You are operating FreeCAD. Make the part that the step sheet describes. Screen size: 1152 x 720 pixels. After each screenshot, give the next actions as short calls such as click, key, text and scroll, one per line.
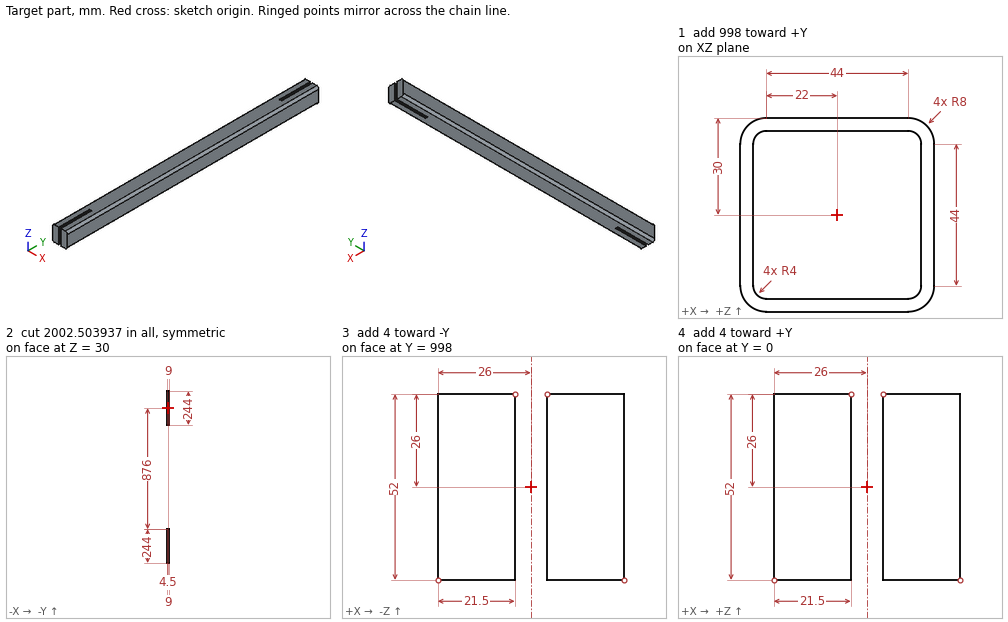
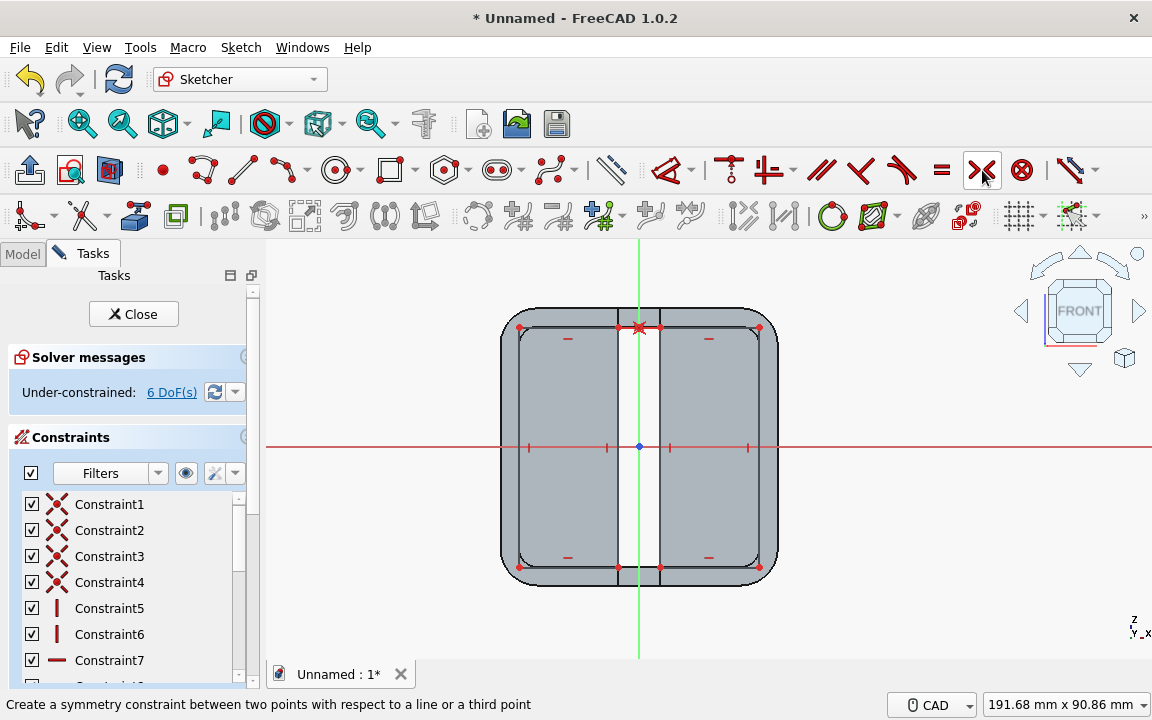
click(519, 568)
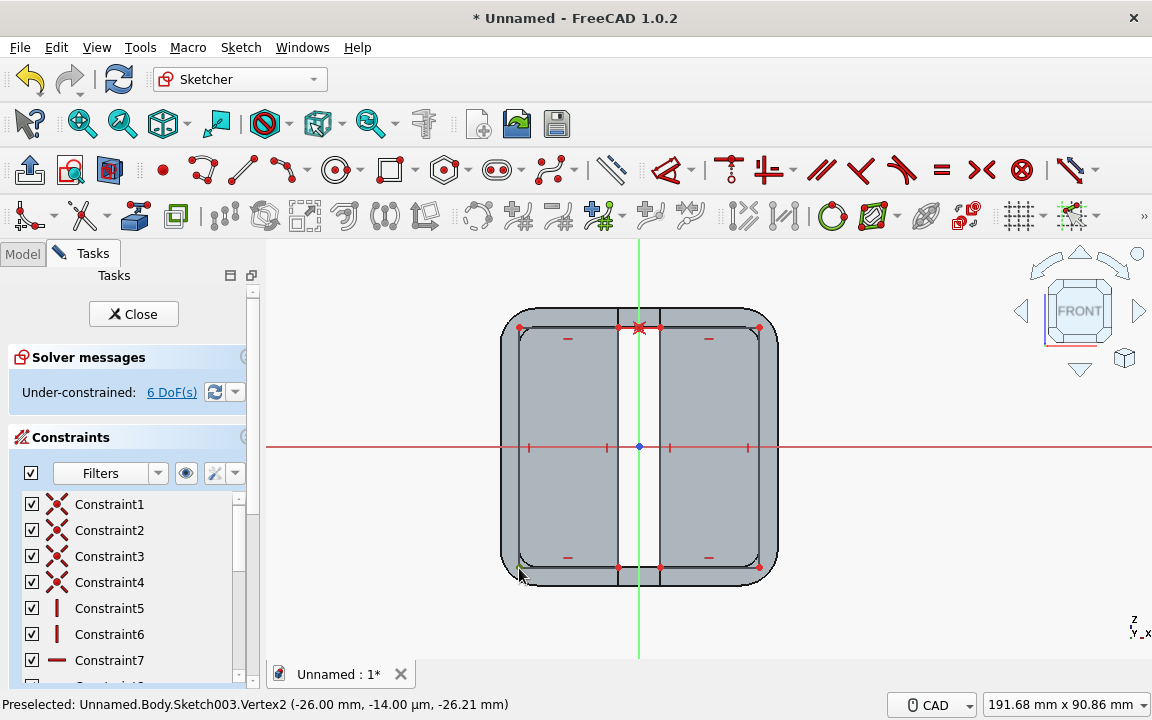
click(759, 568)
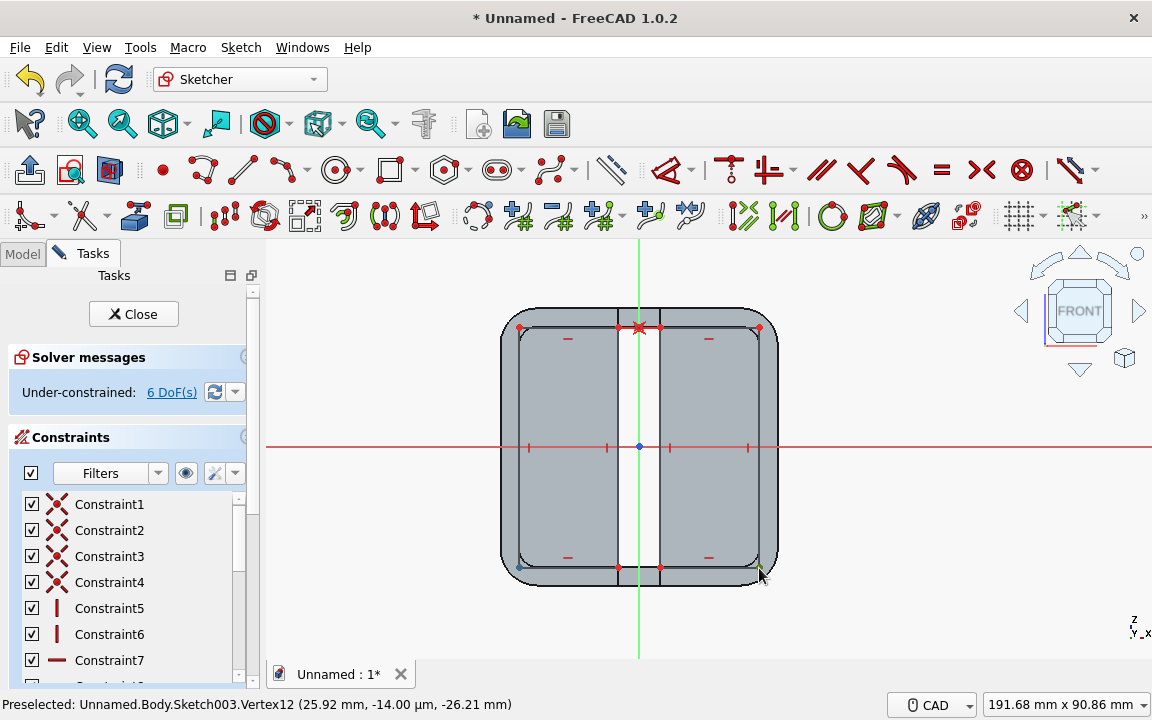
click(639, 605)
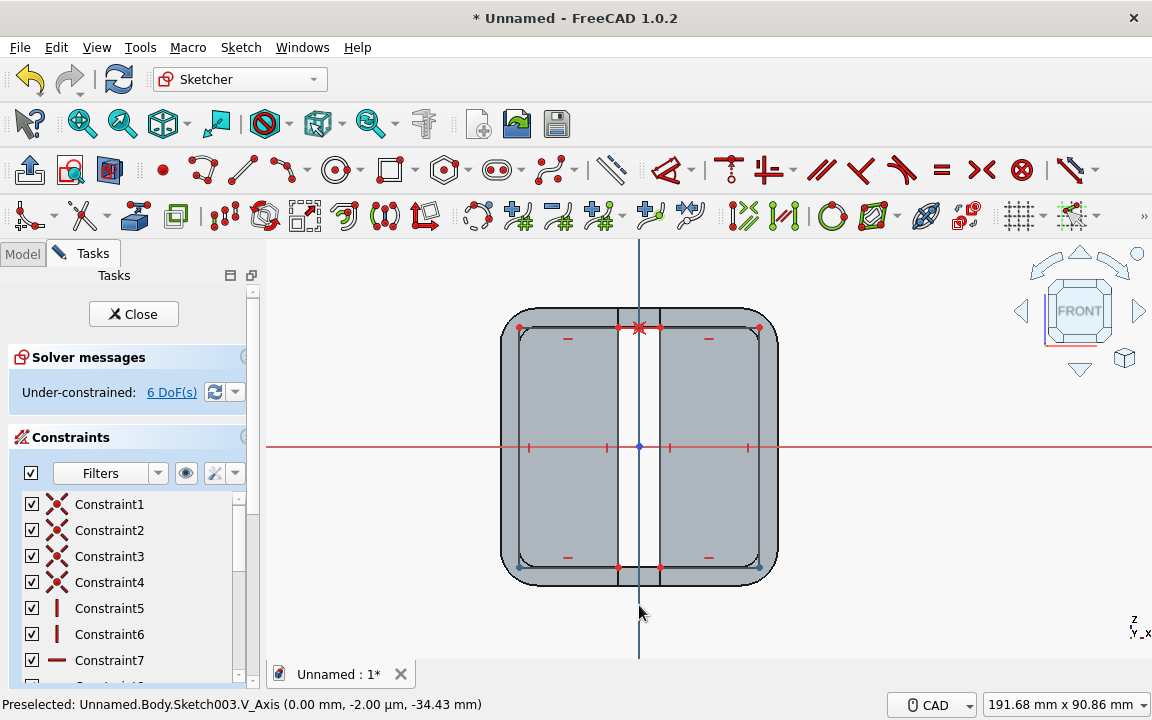
click(982, 170)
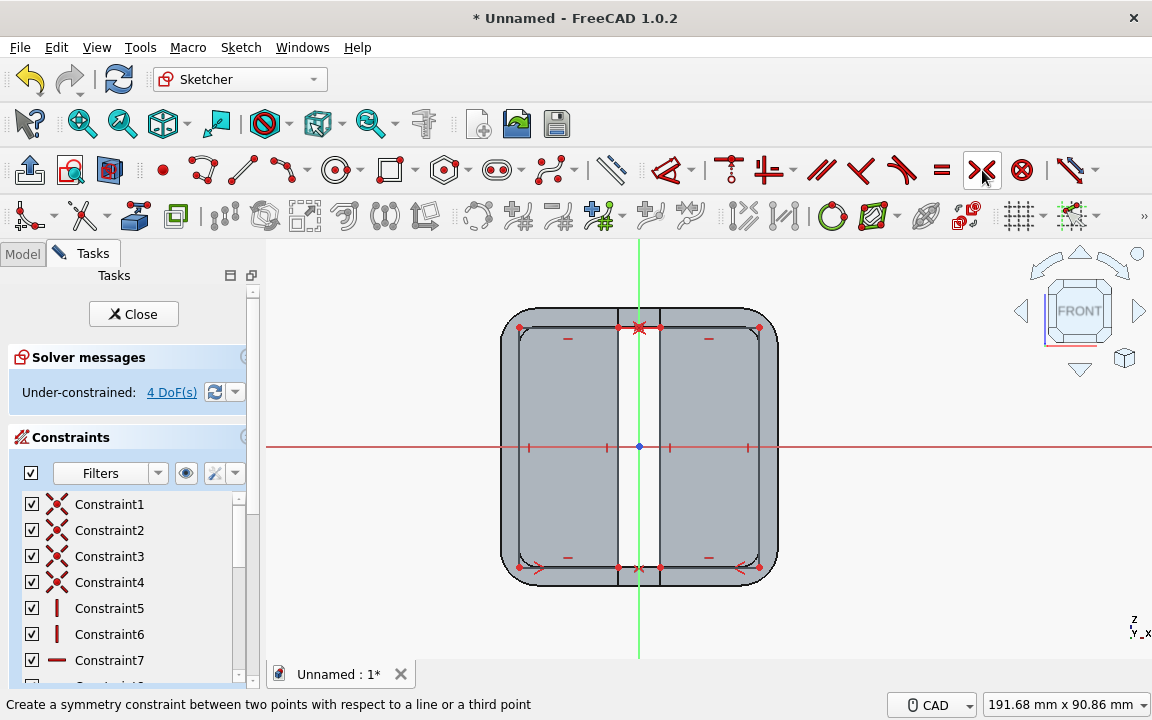
click(666, 170)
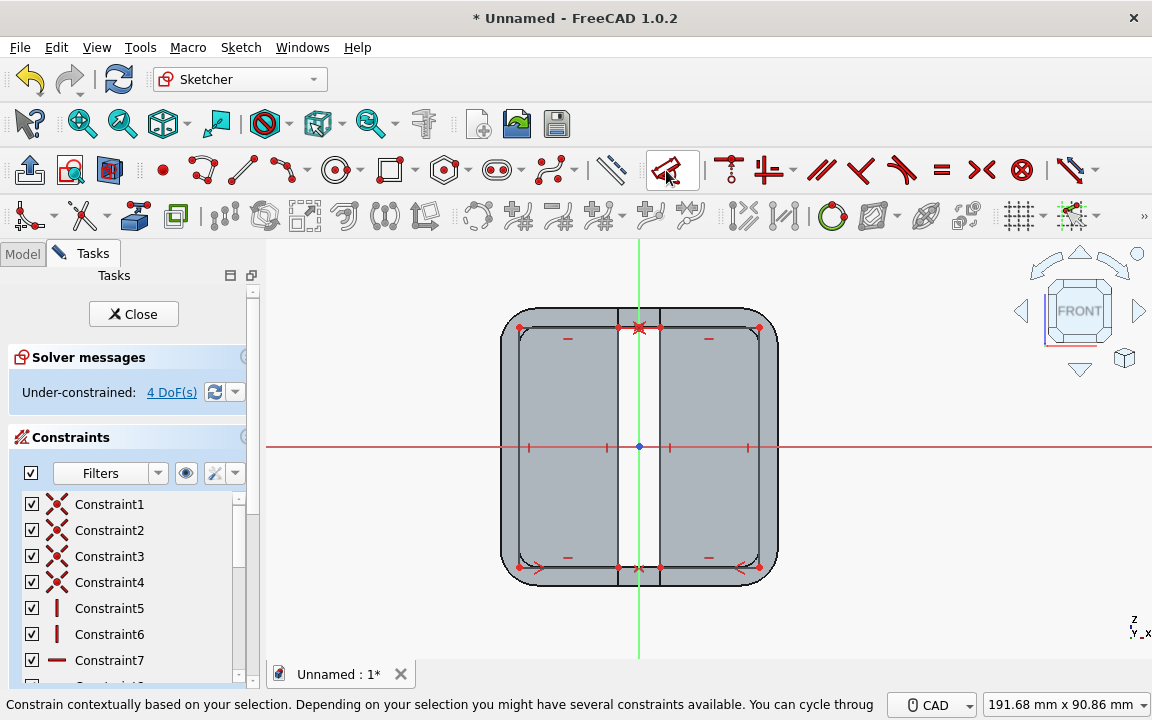
click(519, 400)
click(485, 393)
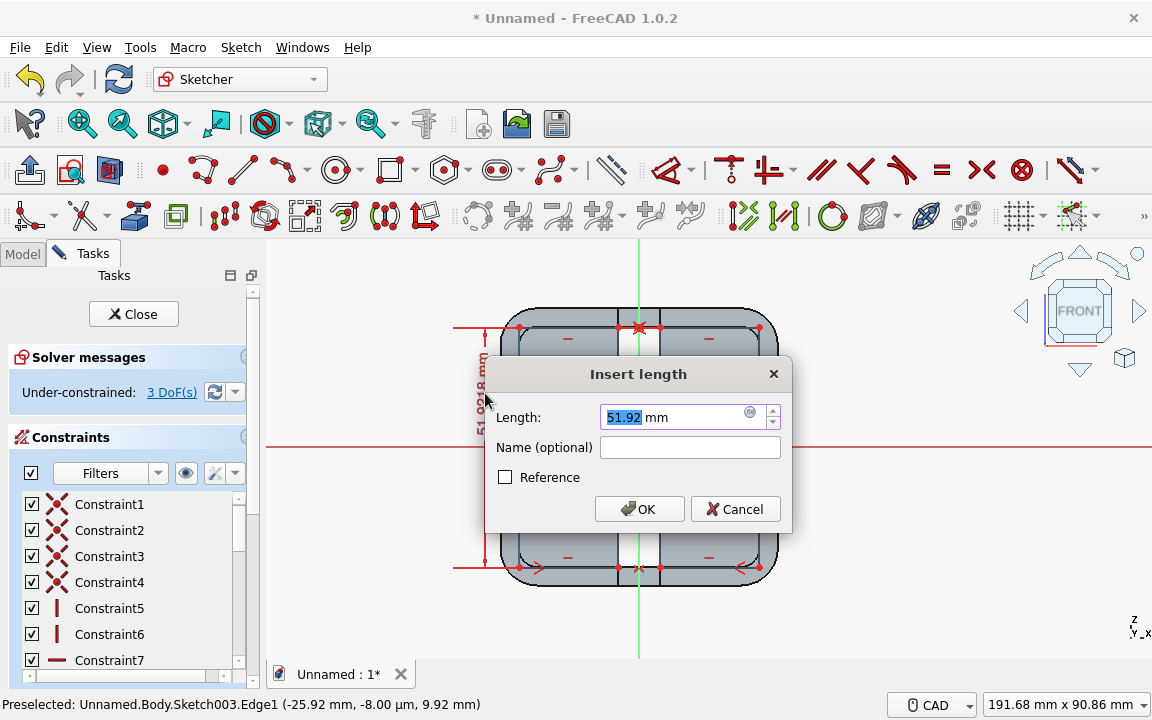
text(52)
key(Return)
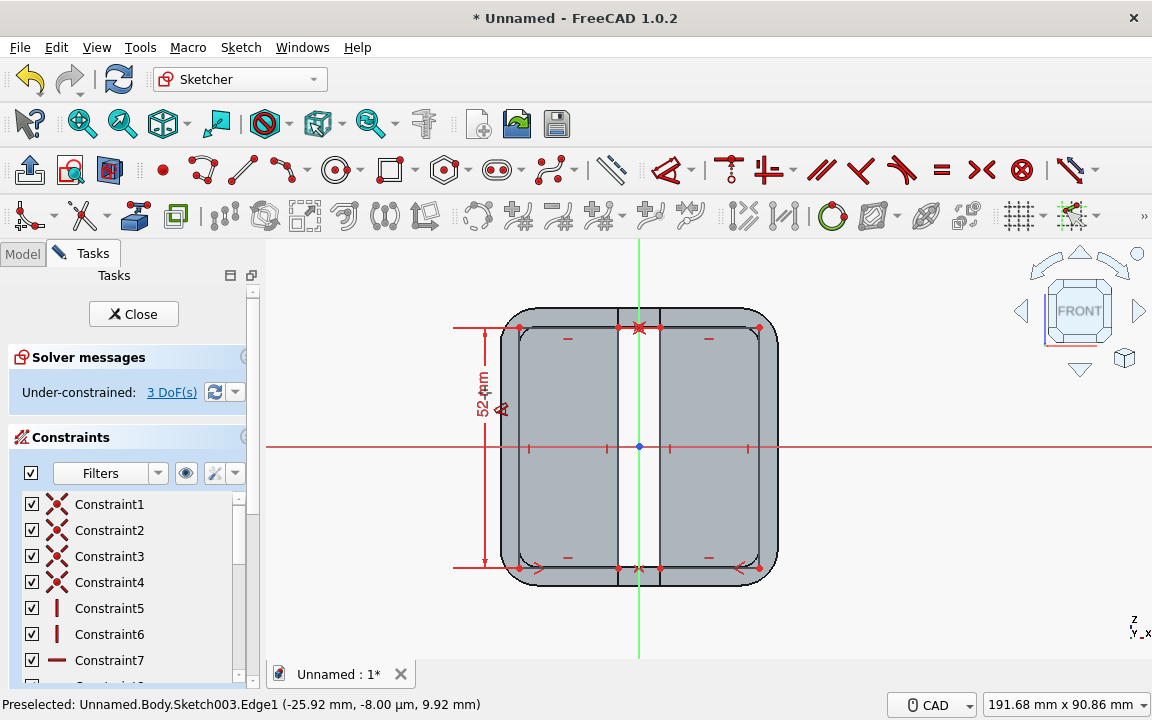
click(519, 328)
click(579, 294)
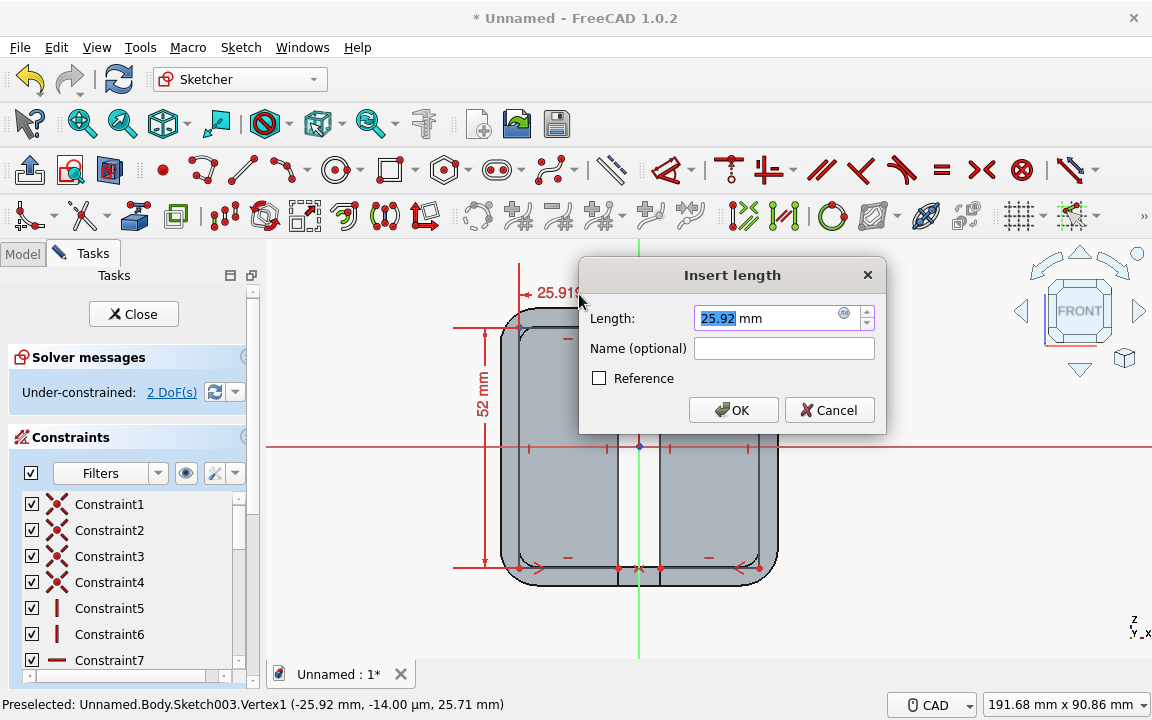
text(26)
key(Return)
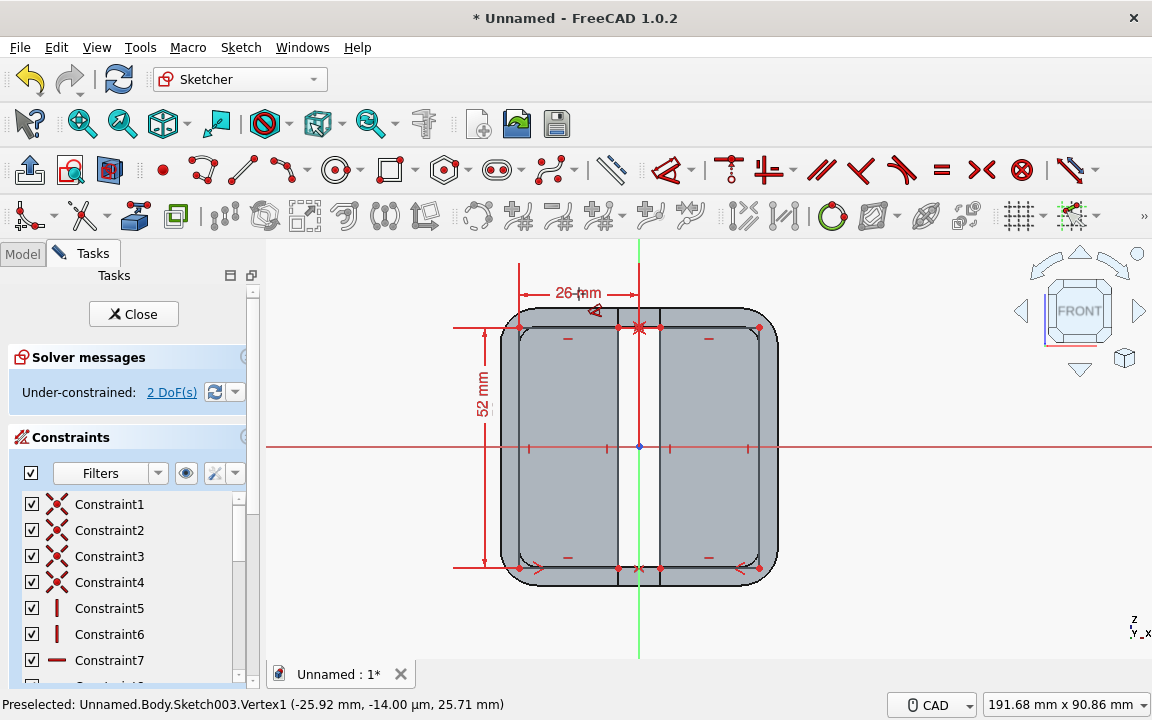
click(519, 328)
click(485, 360)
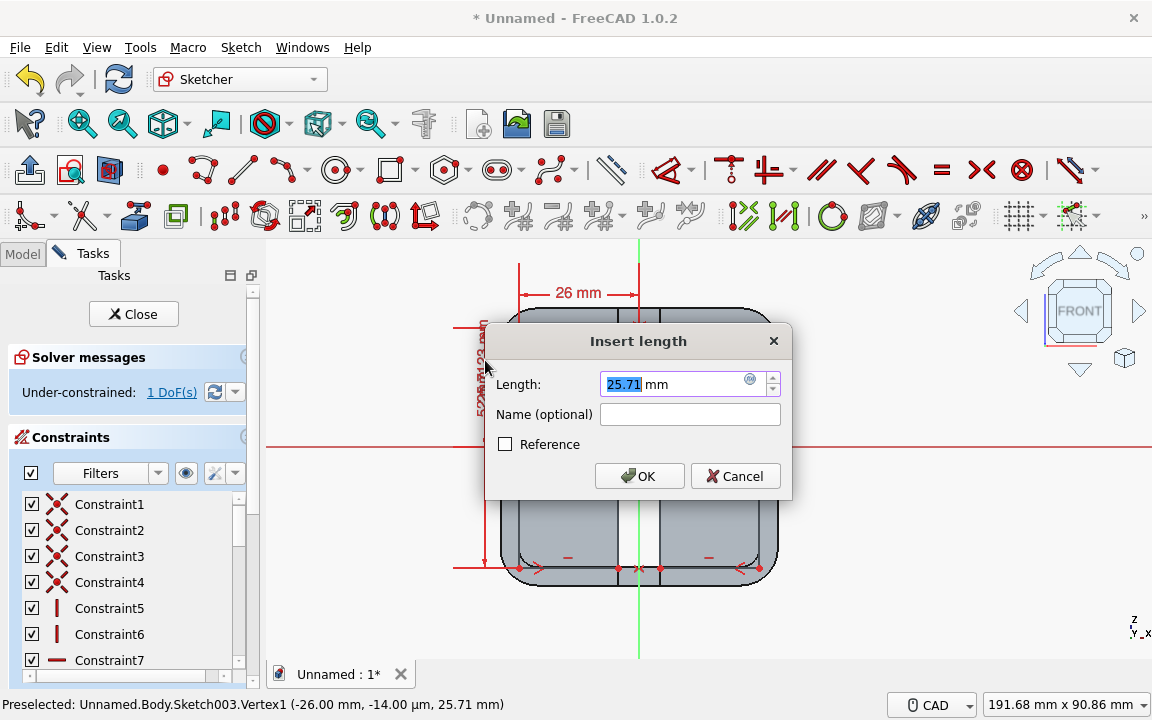
text(26)
key(Return)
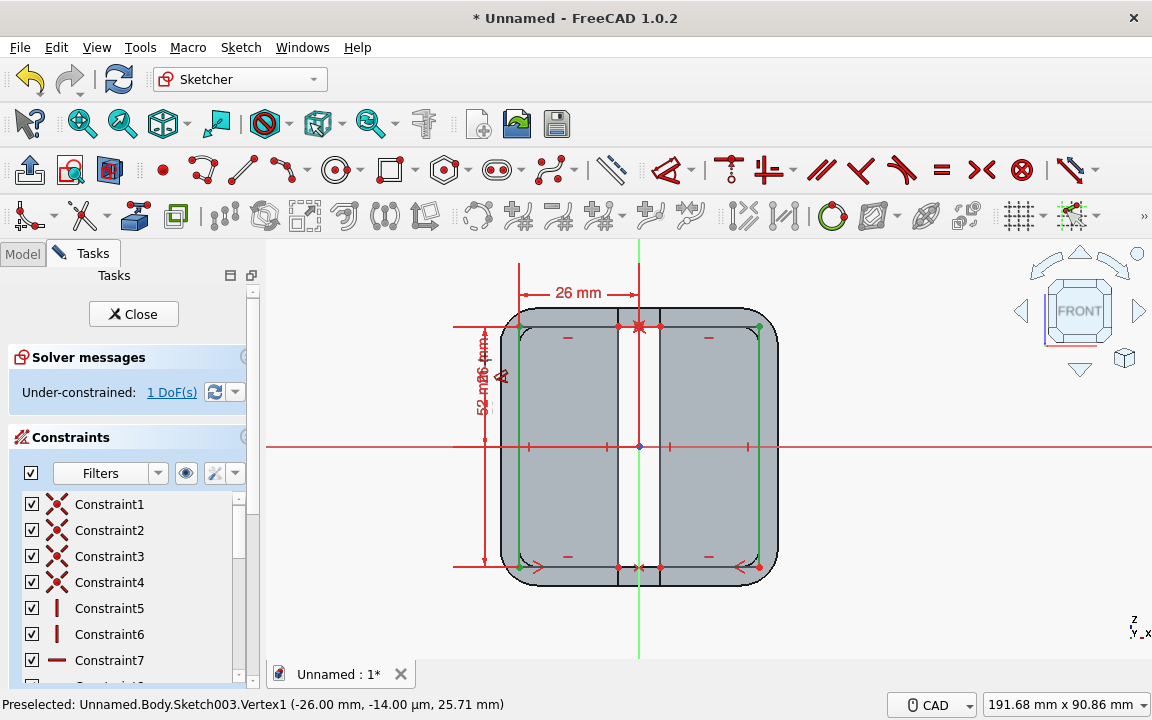
click(549, 567)
click(569, 601)